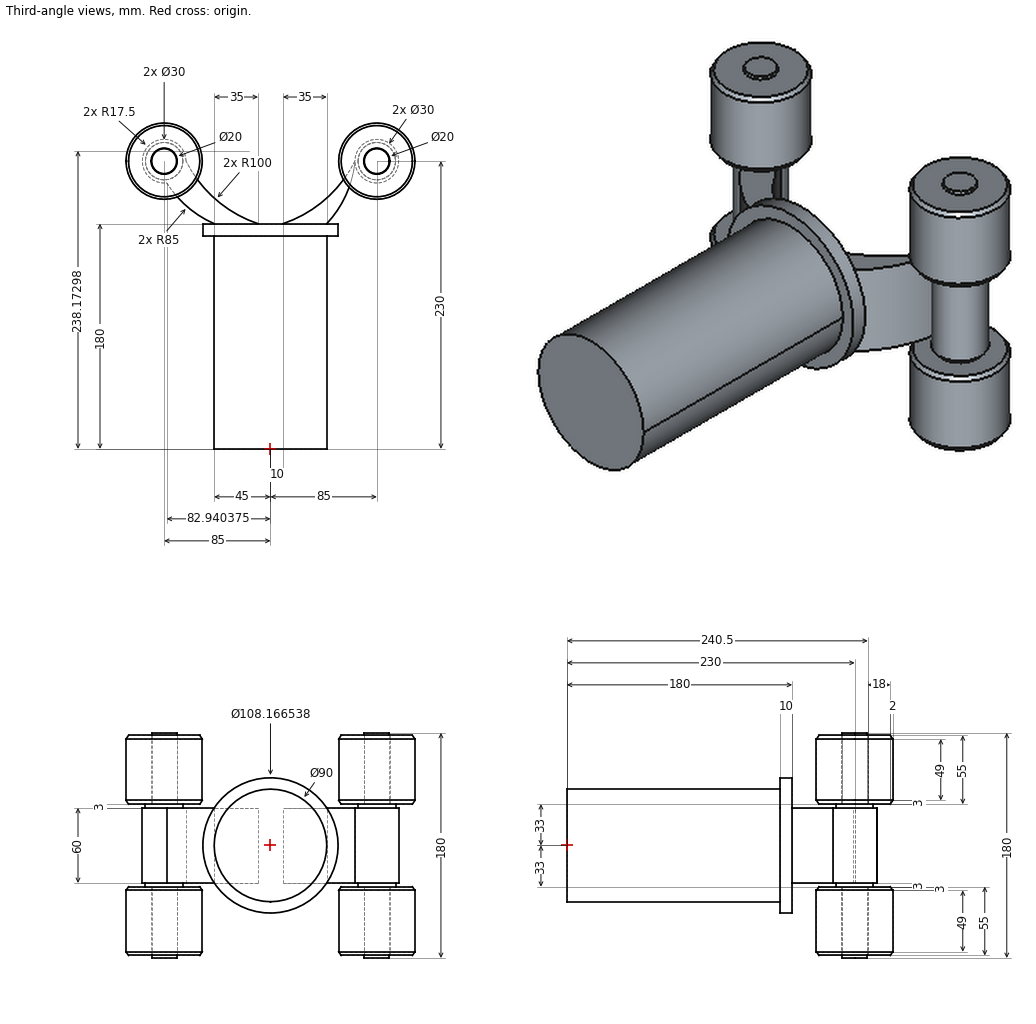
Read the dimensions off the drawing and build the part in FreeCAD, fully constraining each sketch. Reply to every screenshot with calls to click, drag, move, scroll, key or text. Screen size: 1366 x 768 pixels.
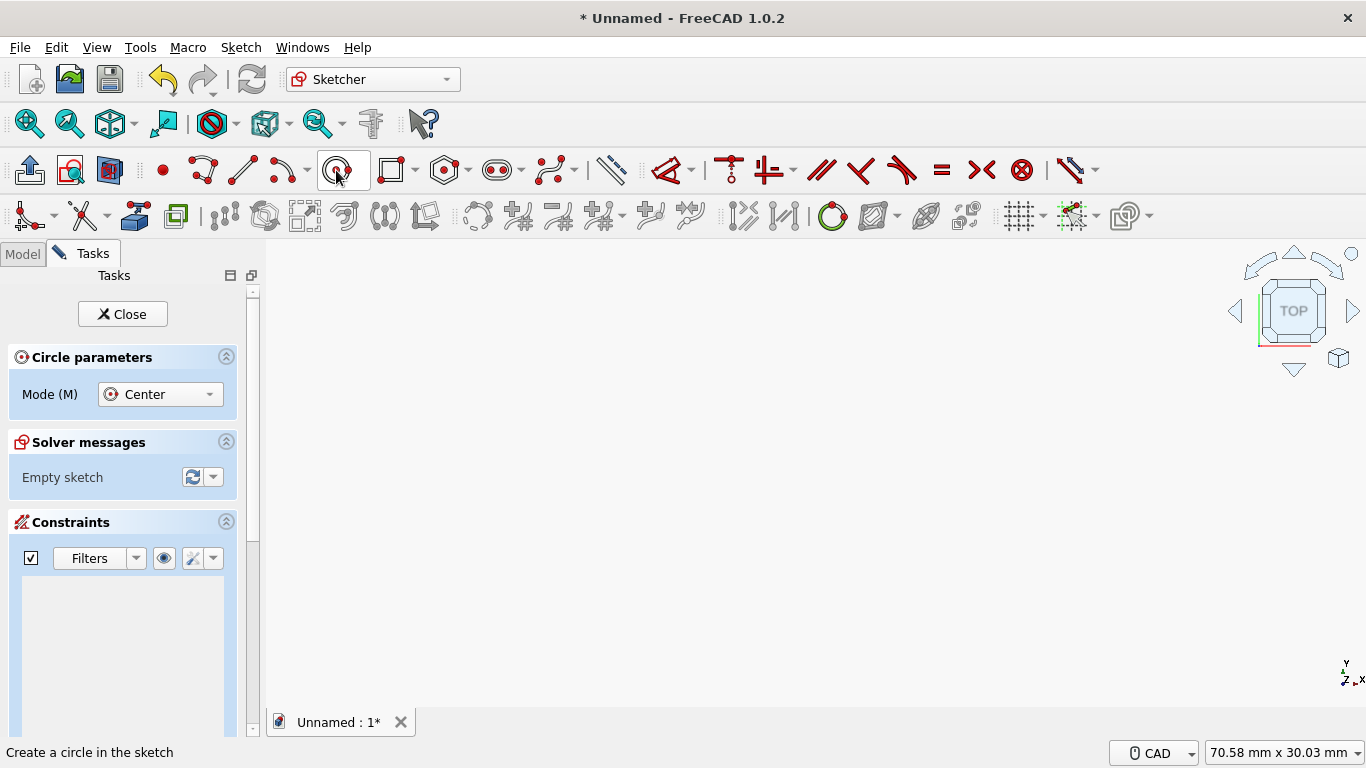
click(742, 471)
click(852, 360)
key(Escape)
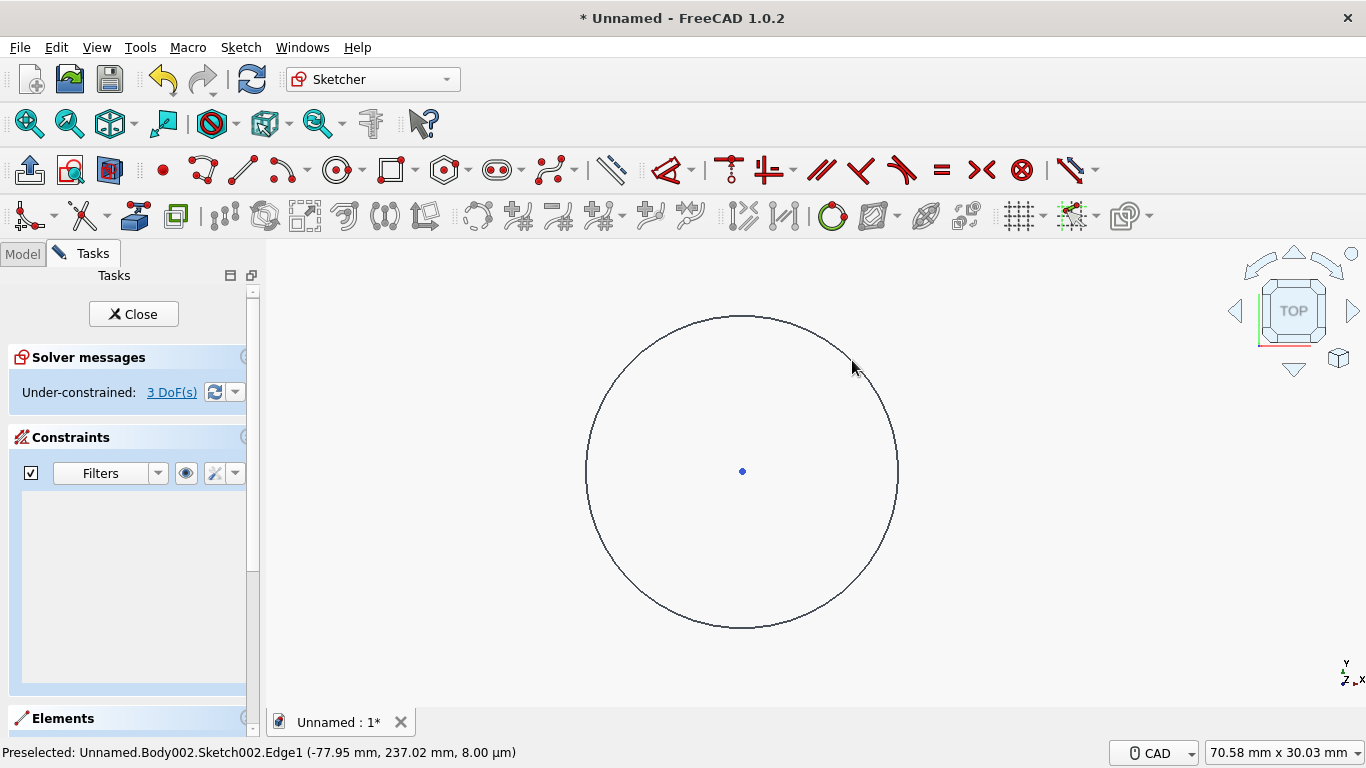
click(666, 170)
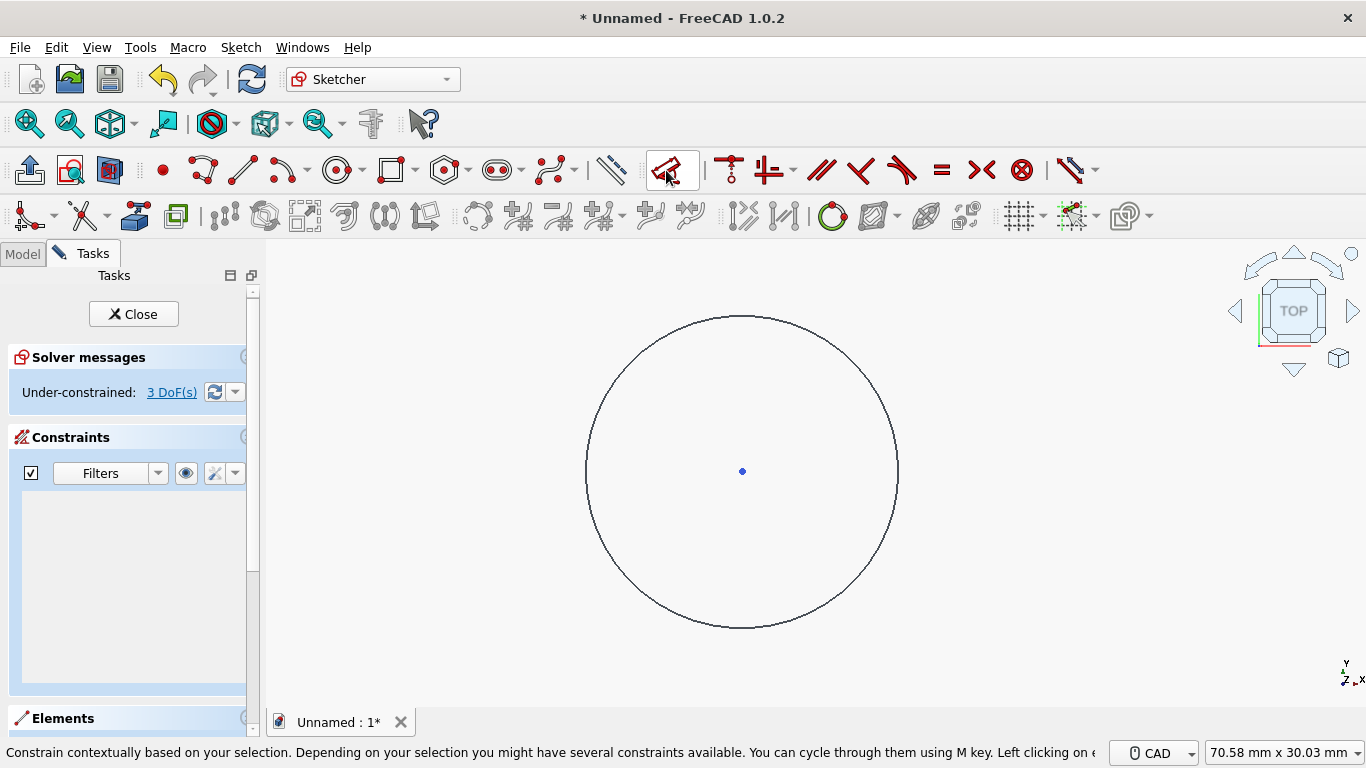
click(852, 361)
click(875, 338)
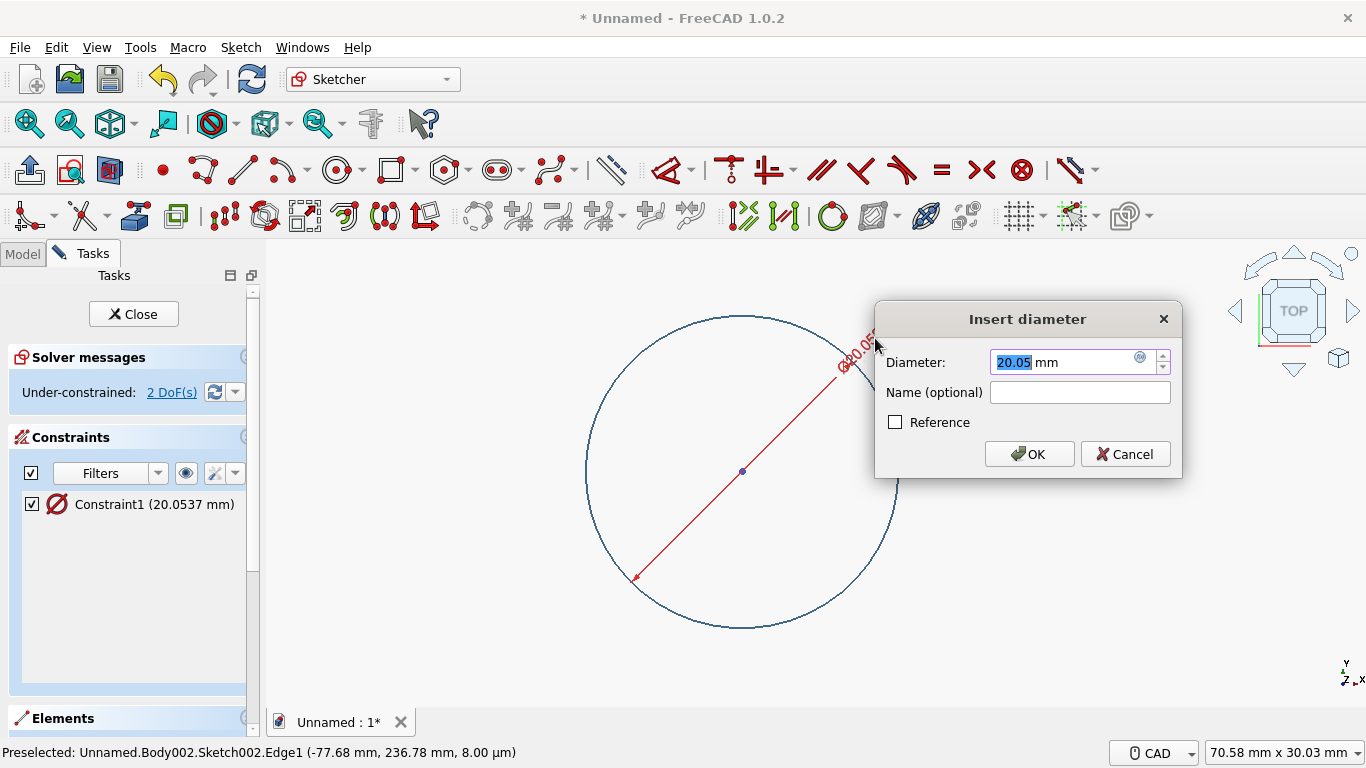
text(20)
key(Return)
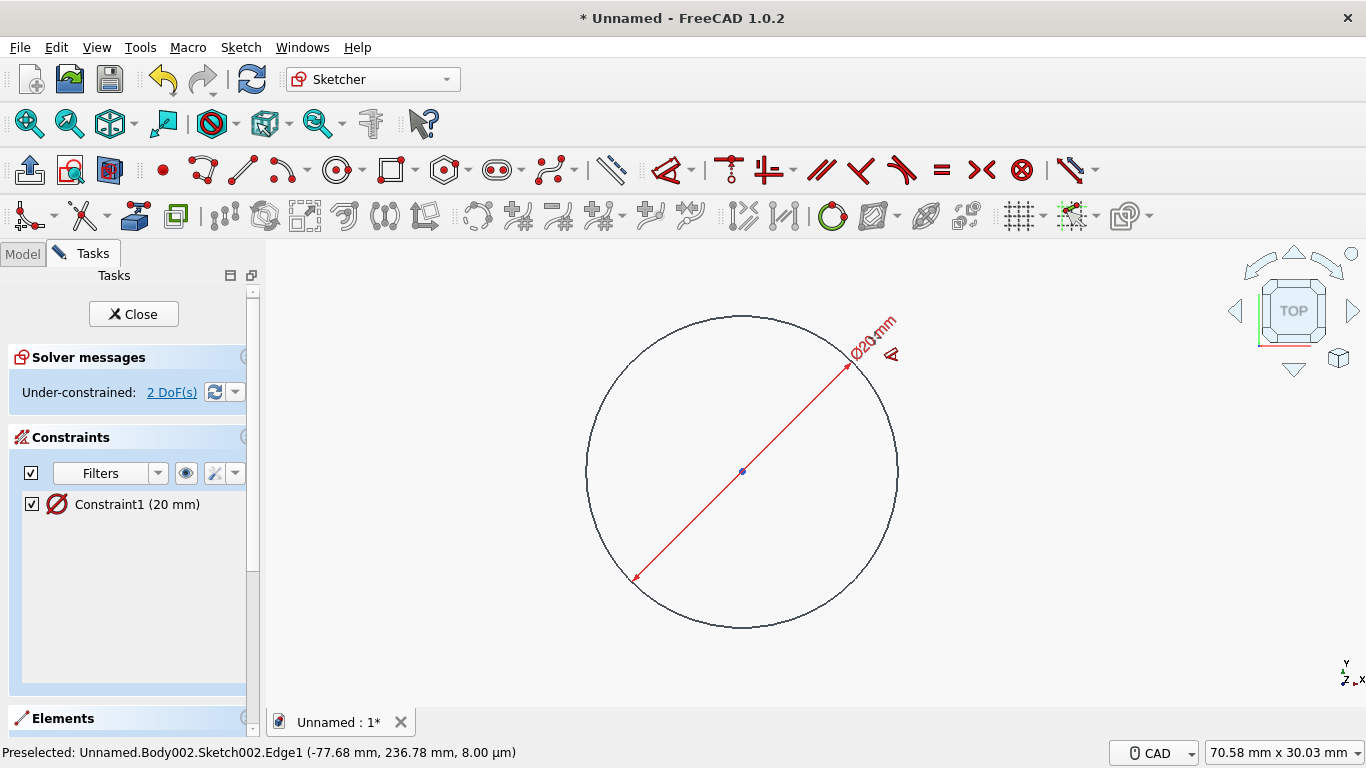
click(742, 472)
click(972, 438)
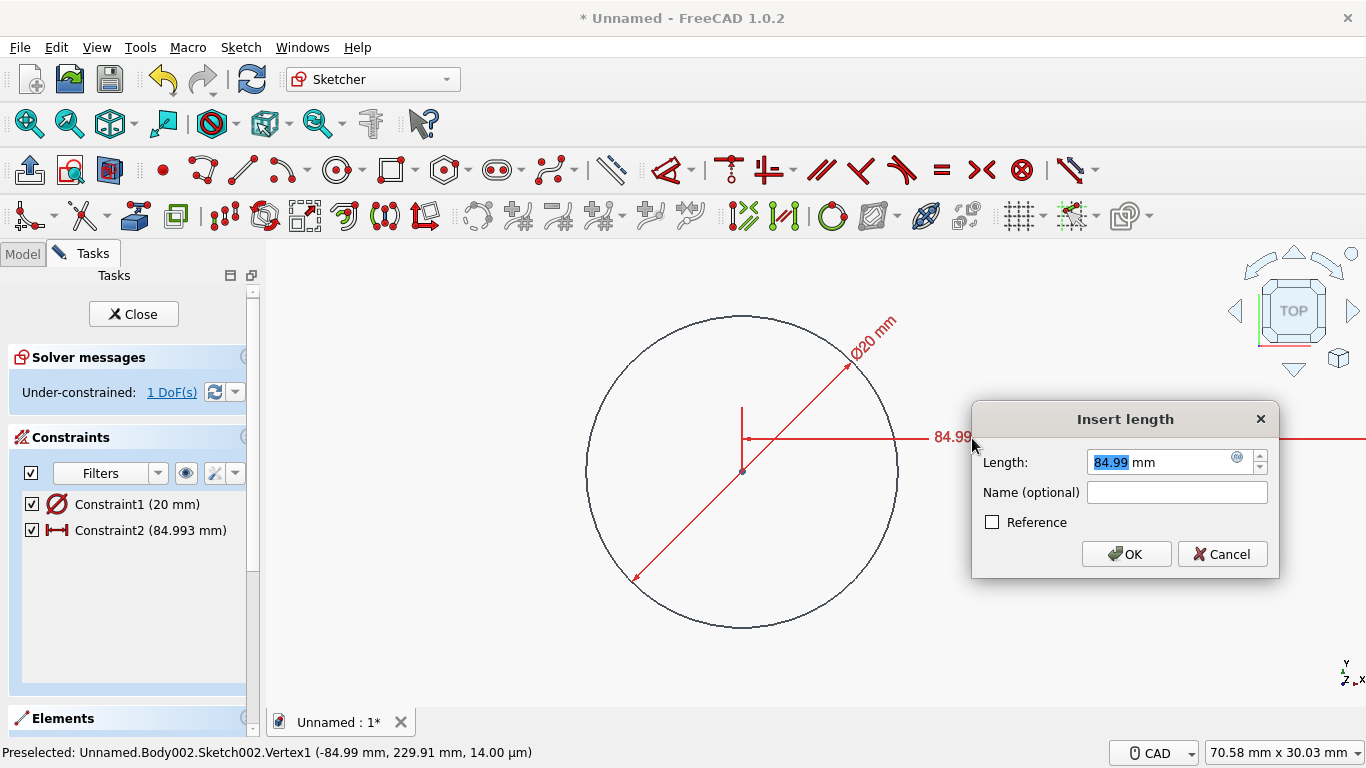
text(85)
key(Return)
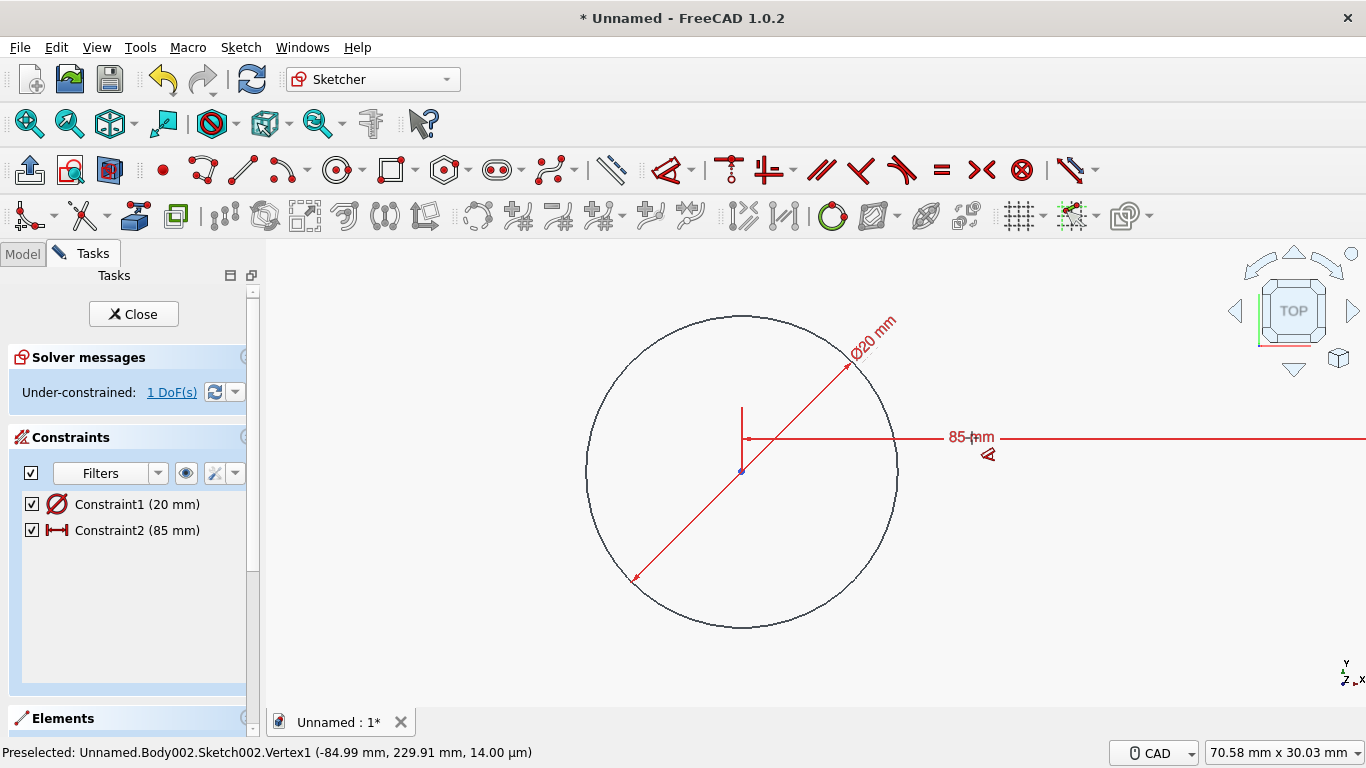
click(742, 472)
click(708, 575)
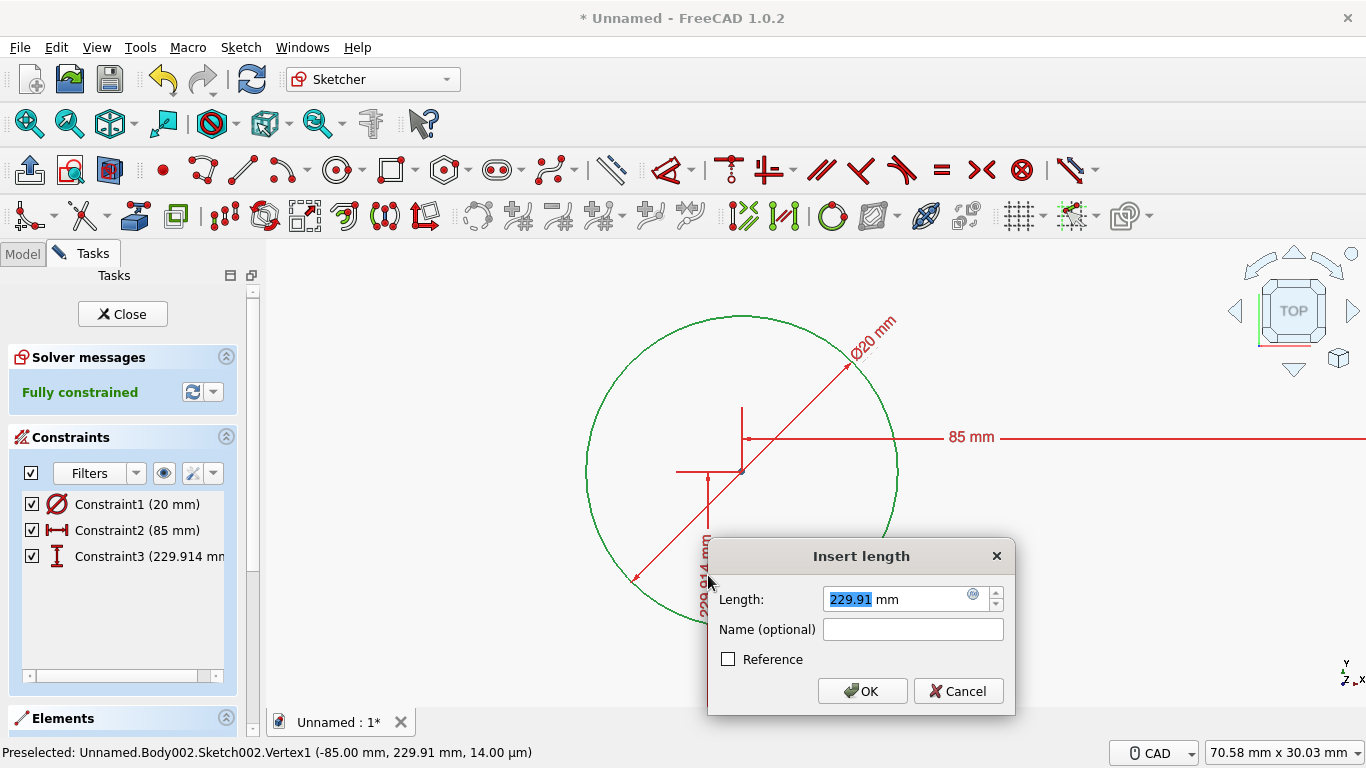
text(230)
key(Return)
key(Escape)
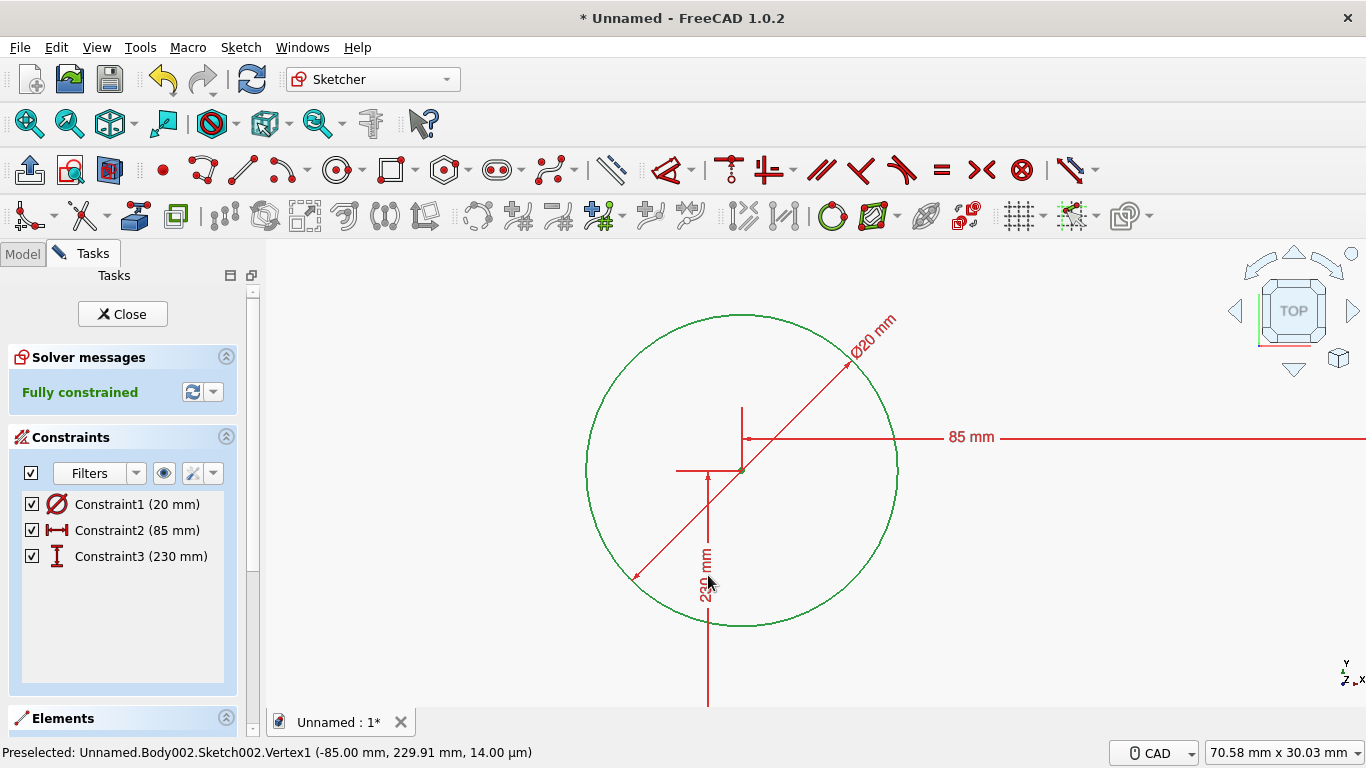
click(123, 314)